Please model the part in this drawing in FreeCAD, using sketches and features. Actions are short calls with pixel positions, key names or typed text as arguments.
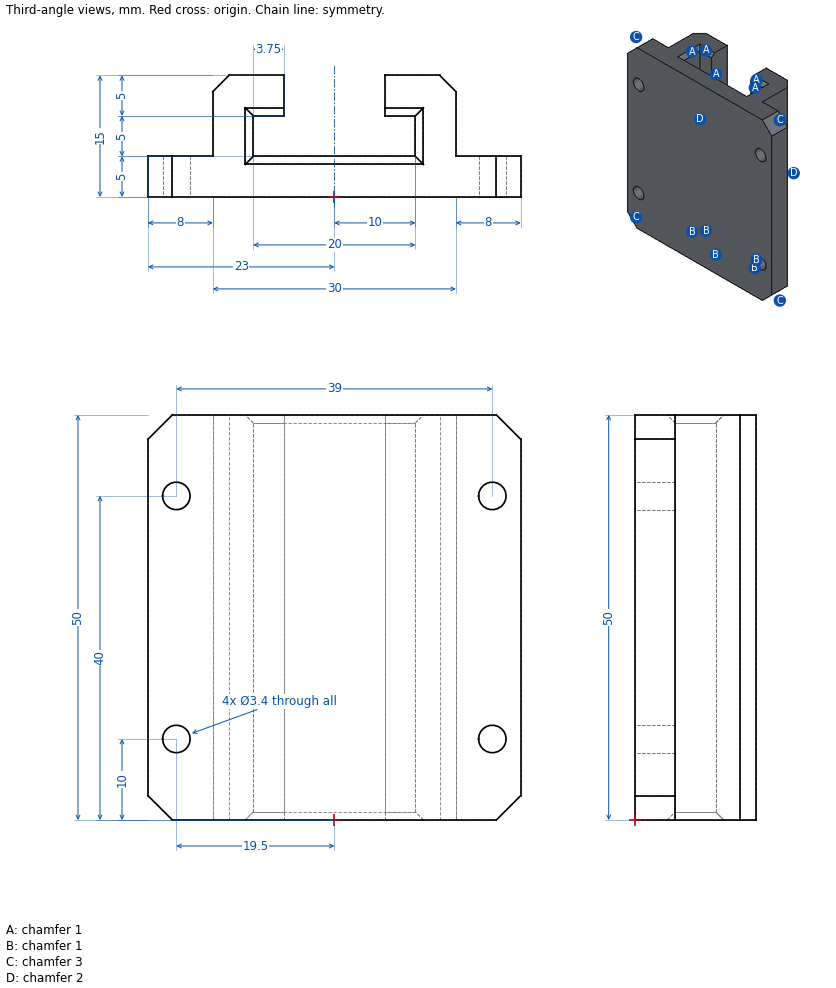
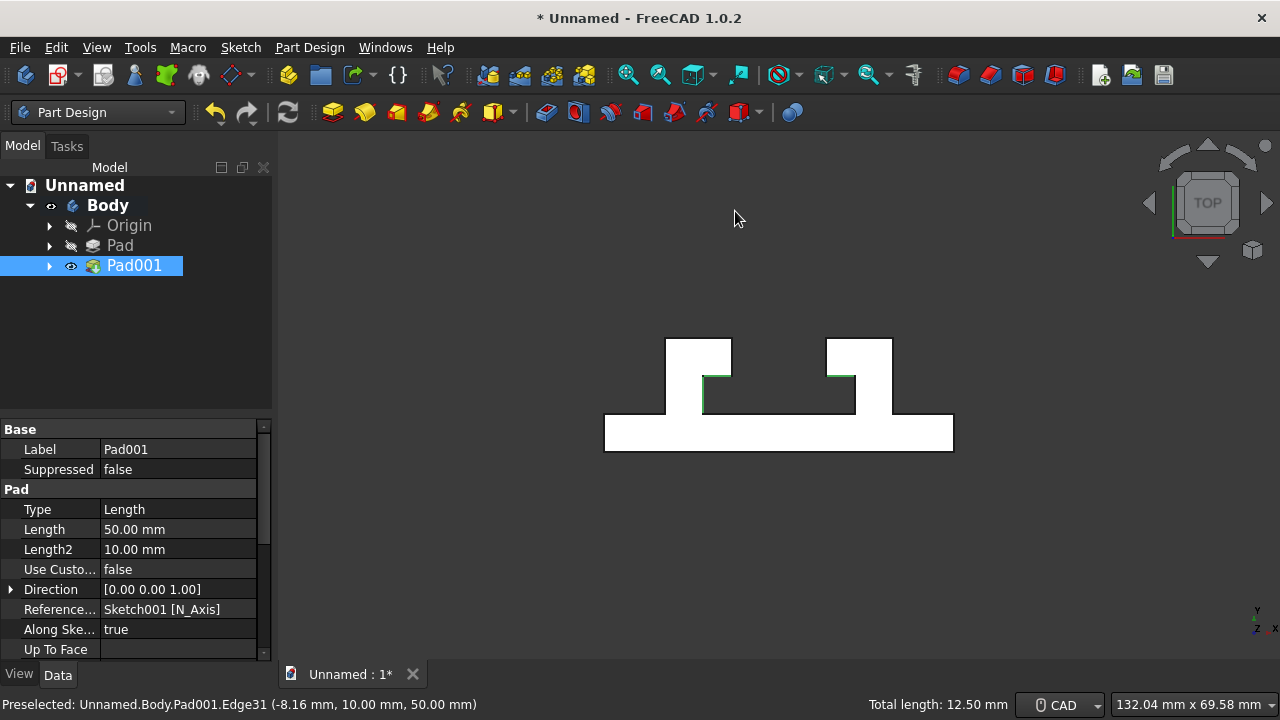
click(855, 394, ctrl)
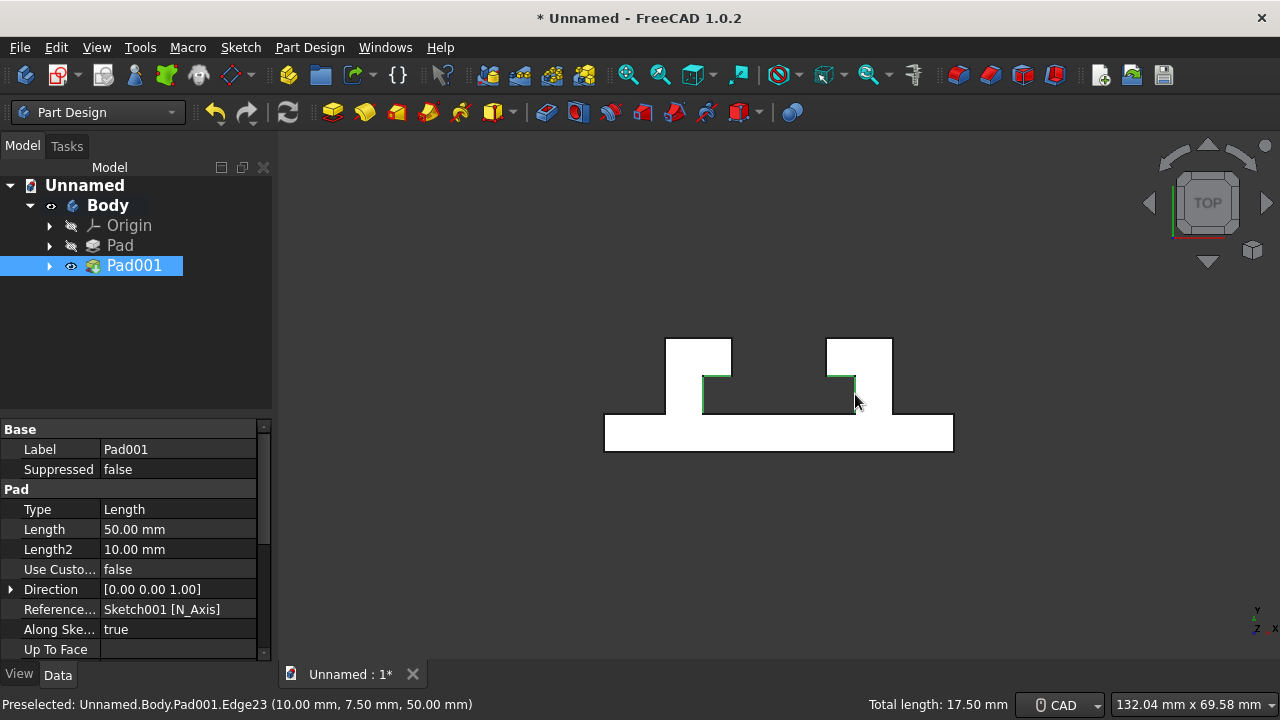
click(779, 413, ctrl)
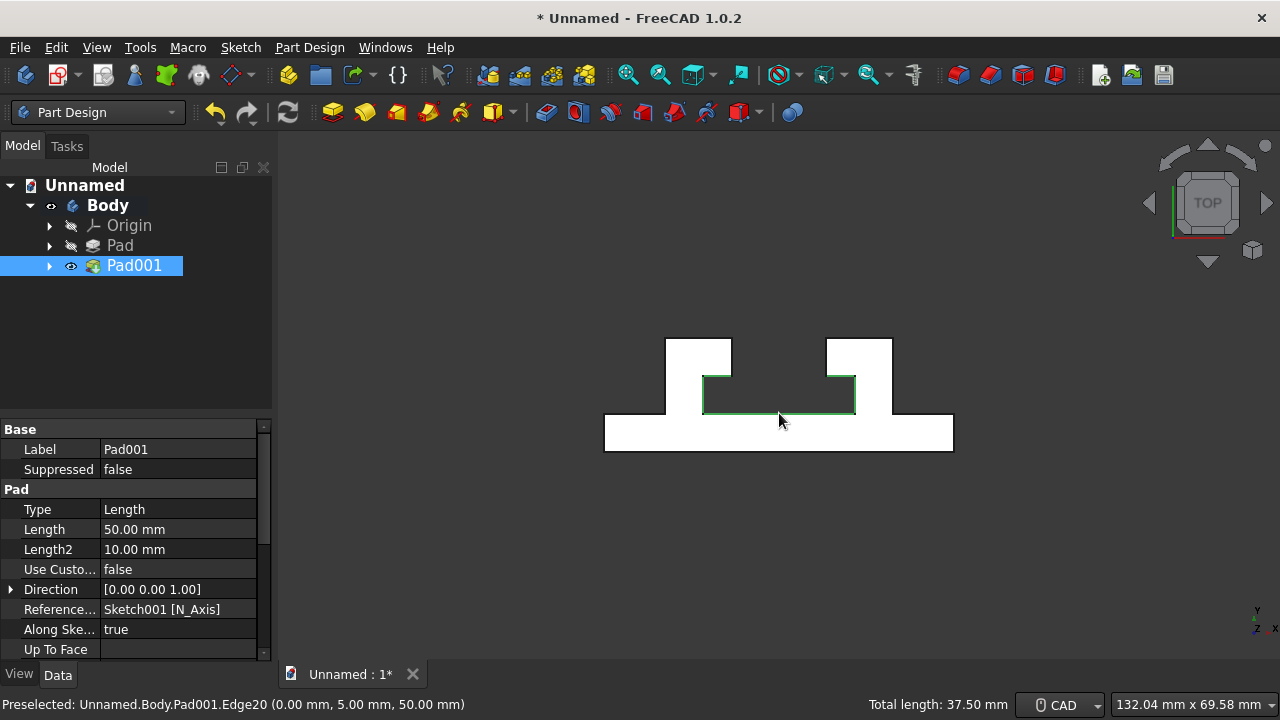
click(992, 76)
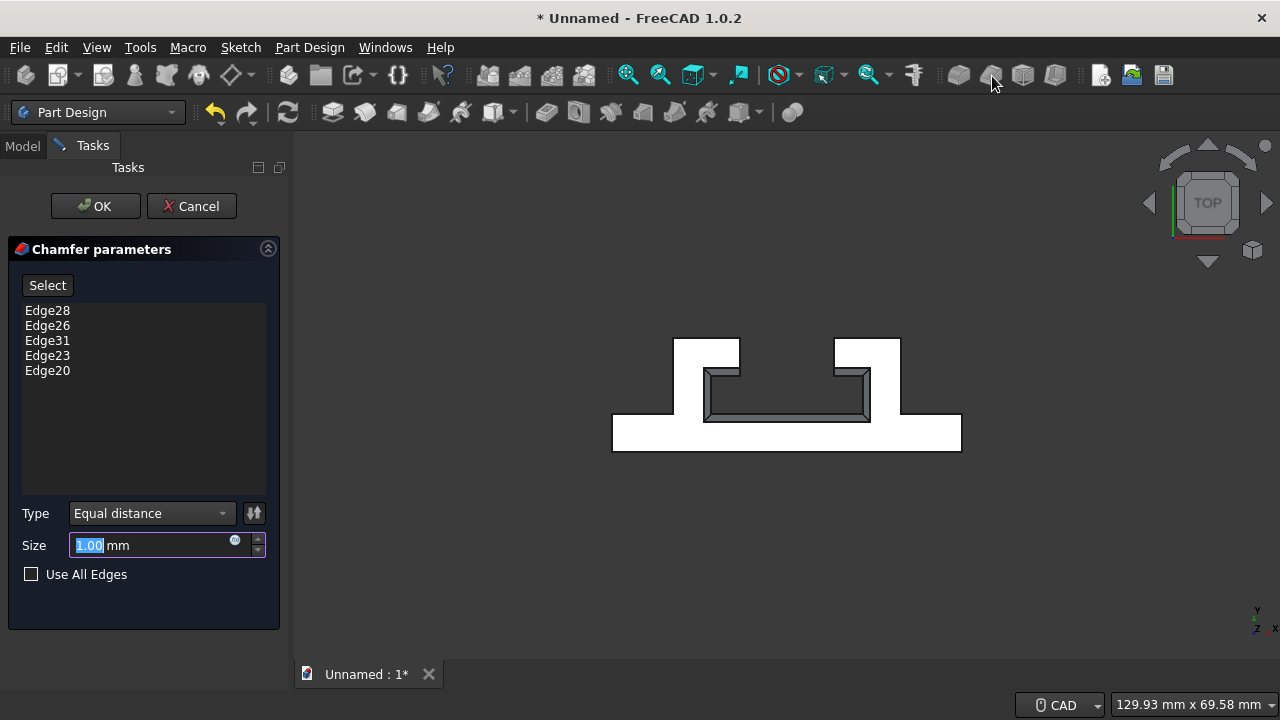
text(1)
key(Tab)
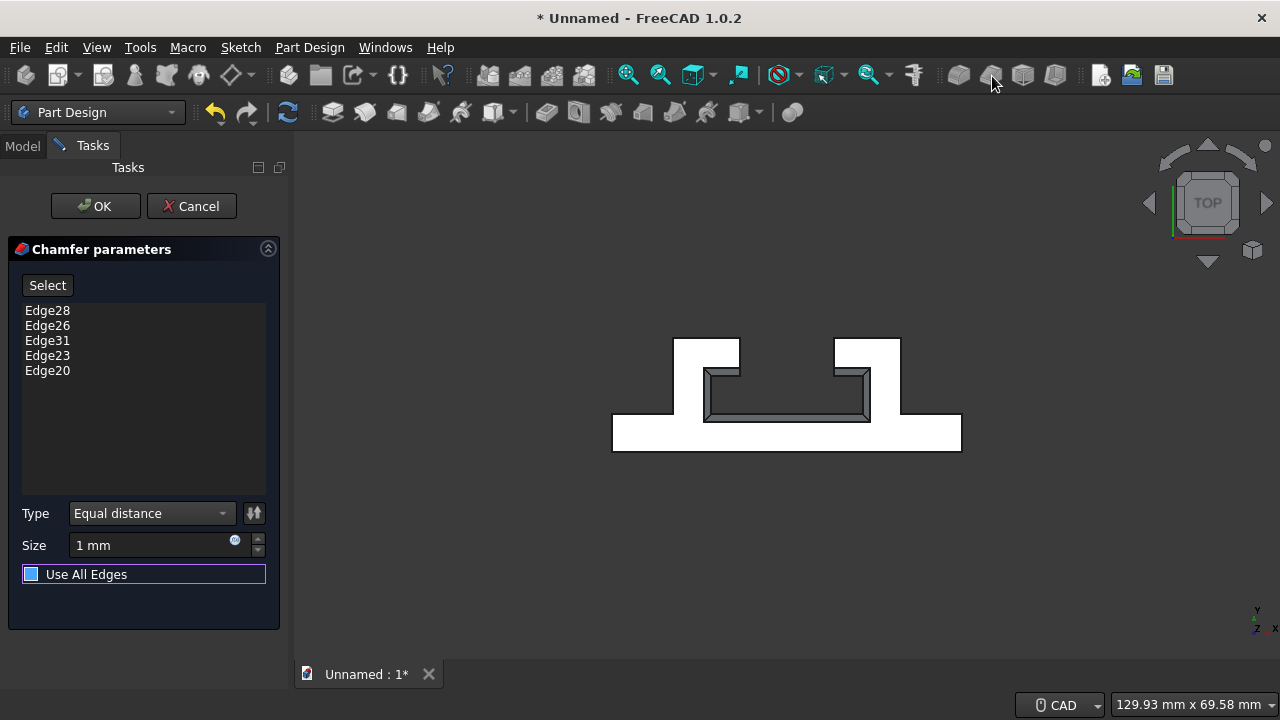
click(96, 206)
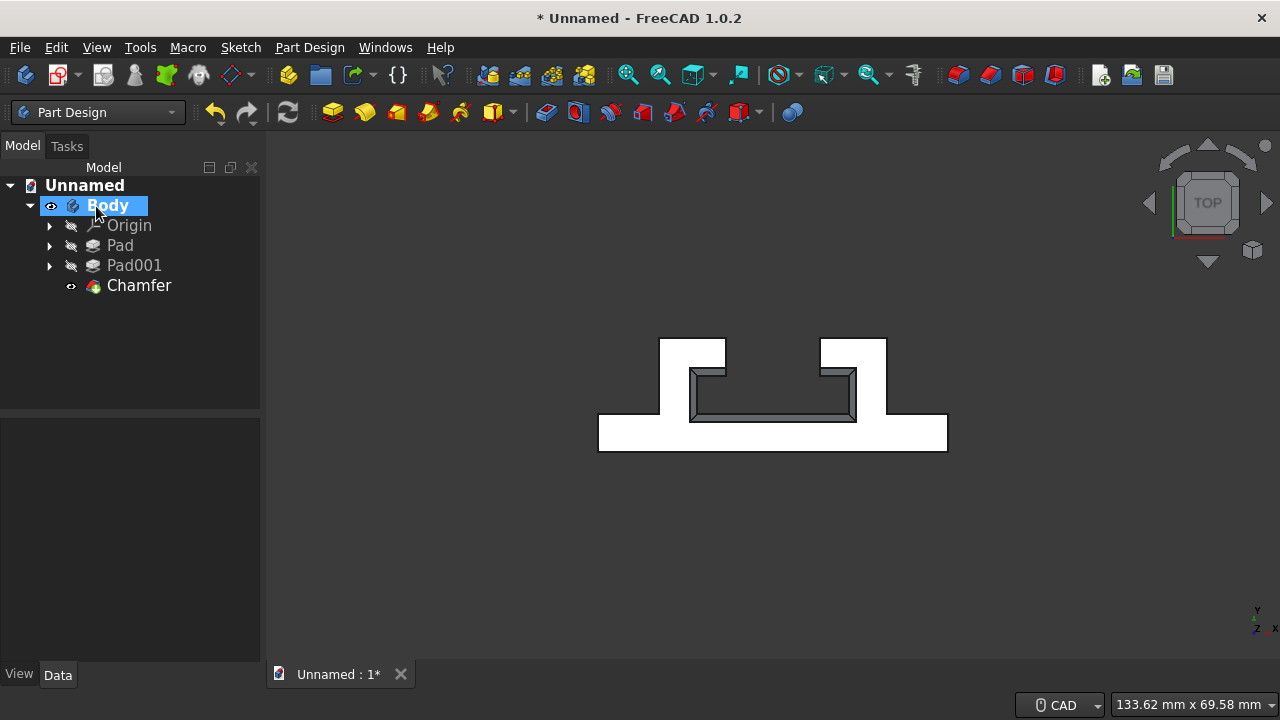
key(v)
key(f)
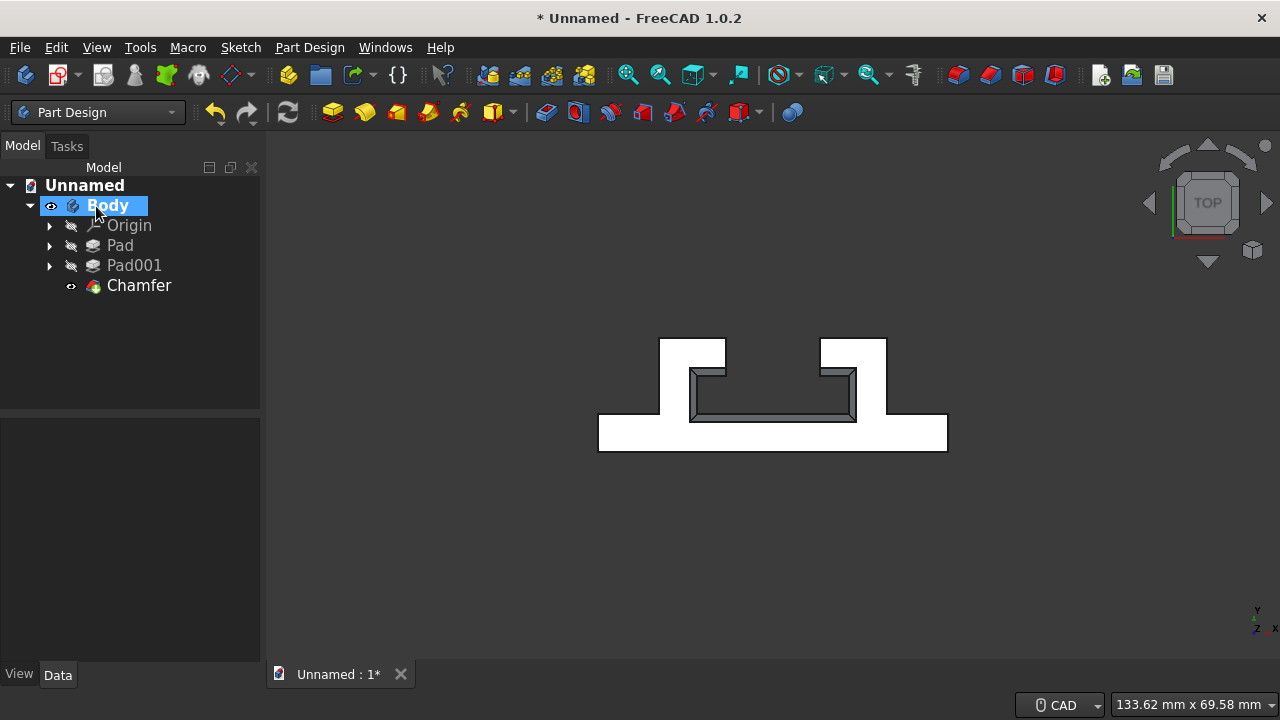
key(0)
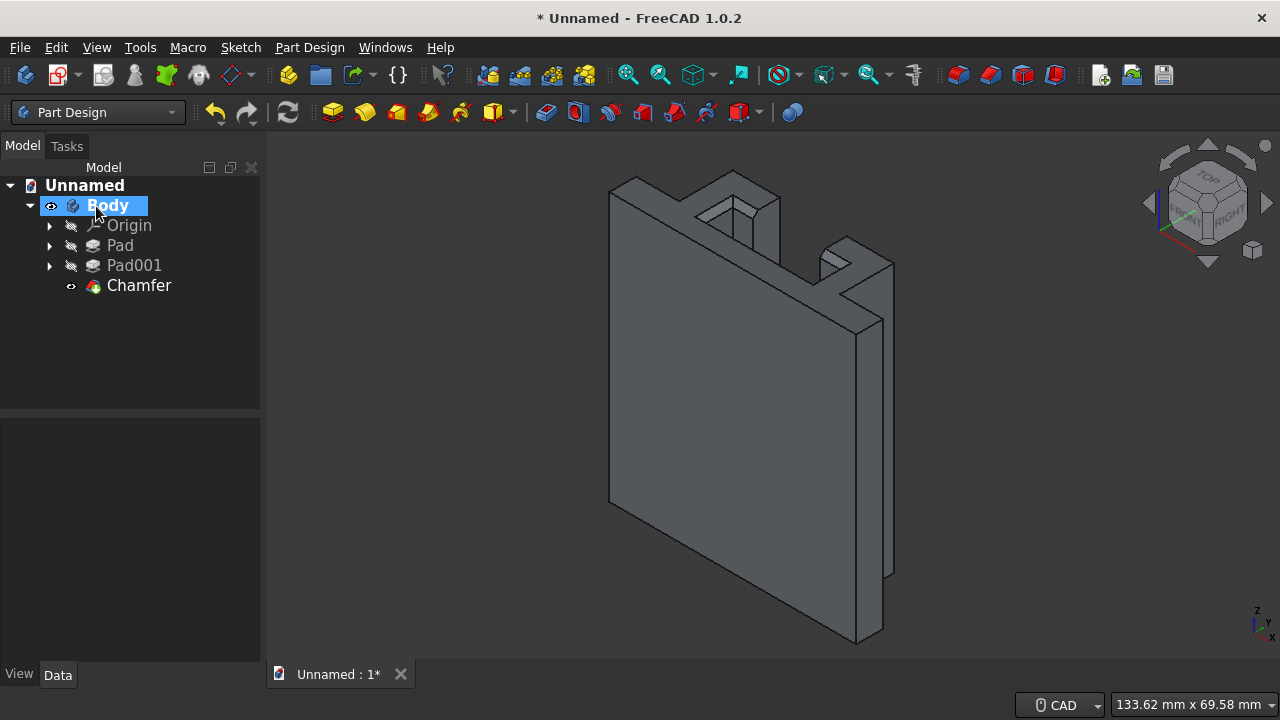
key(2)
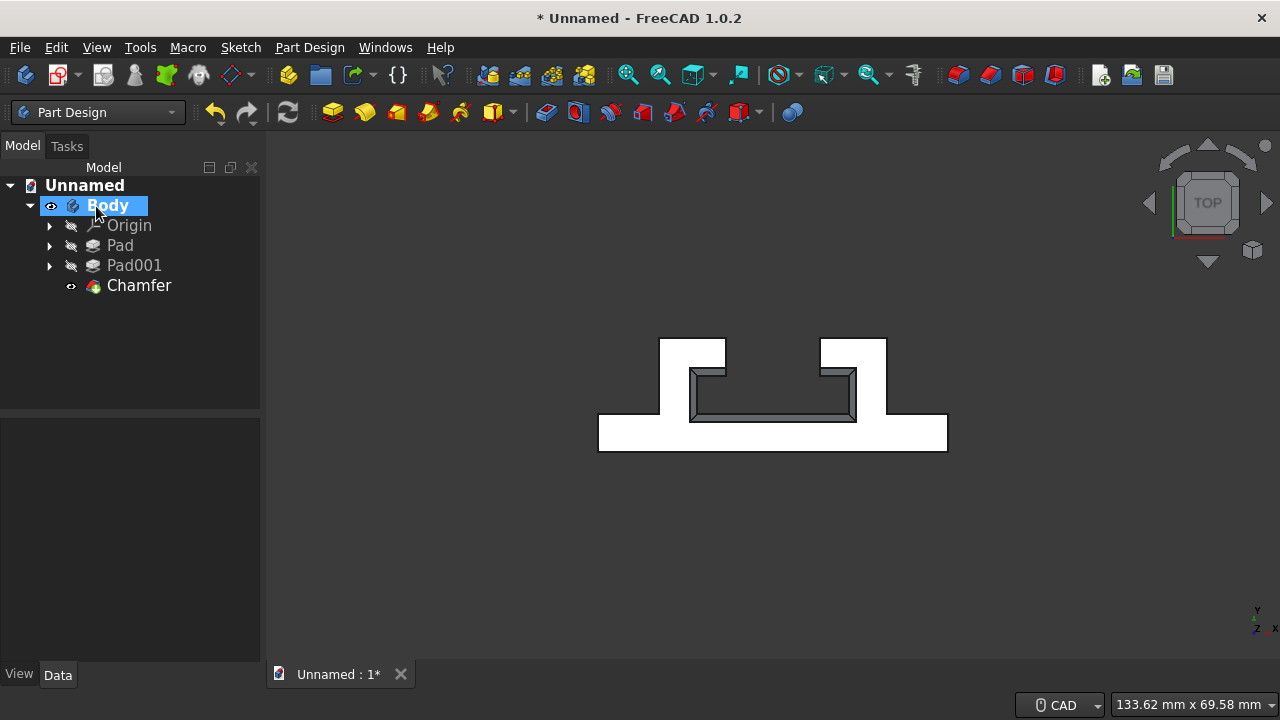
key(v)
key(f)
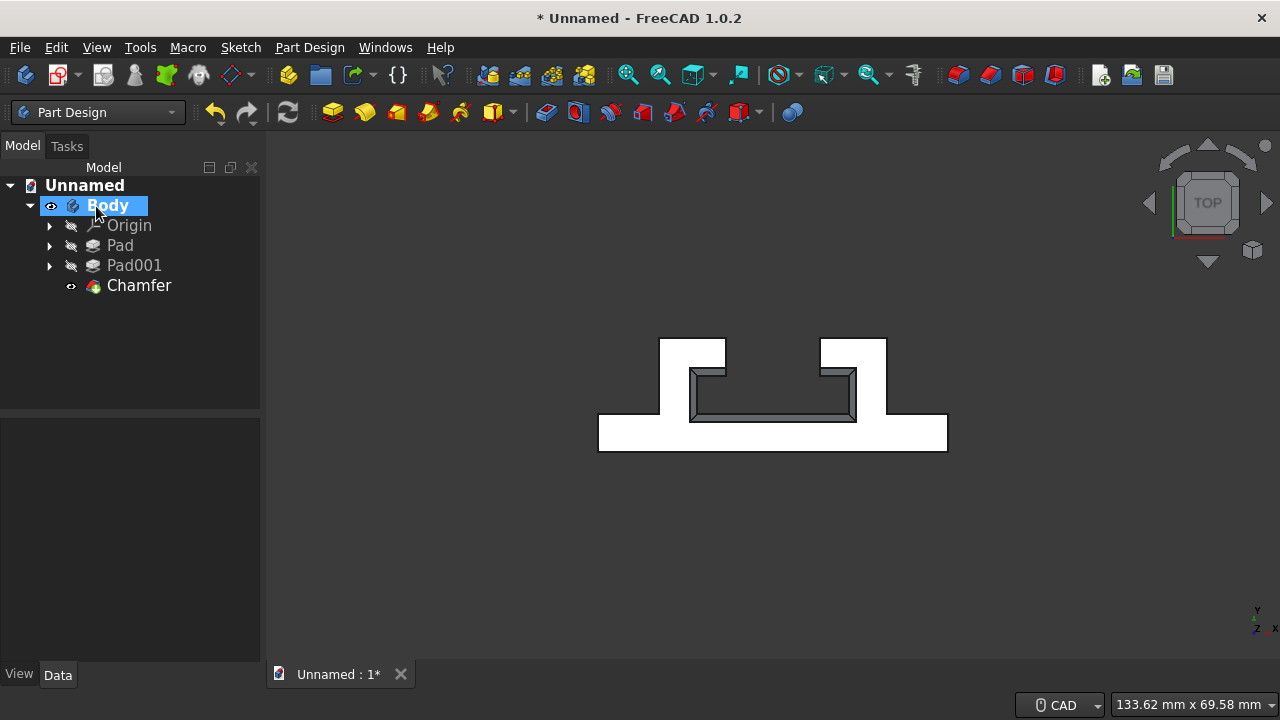
key(1)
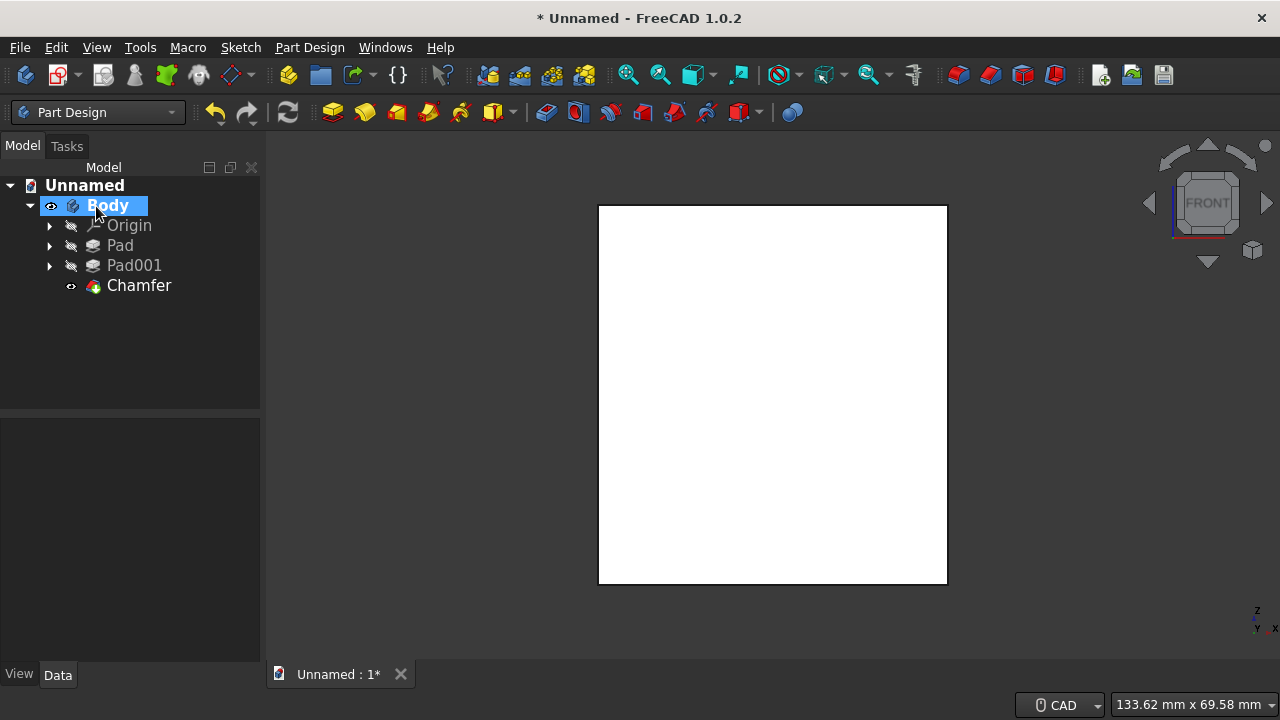
key(3)